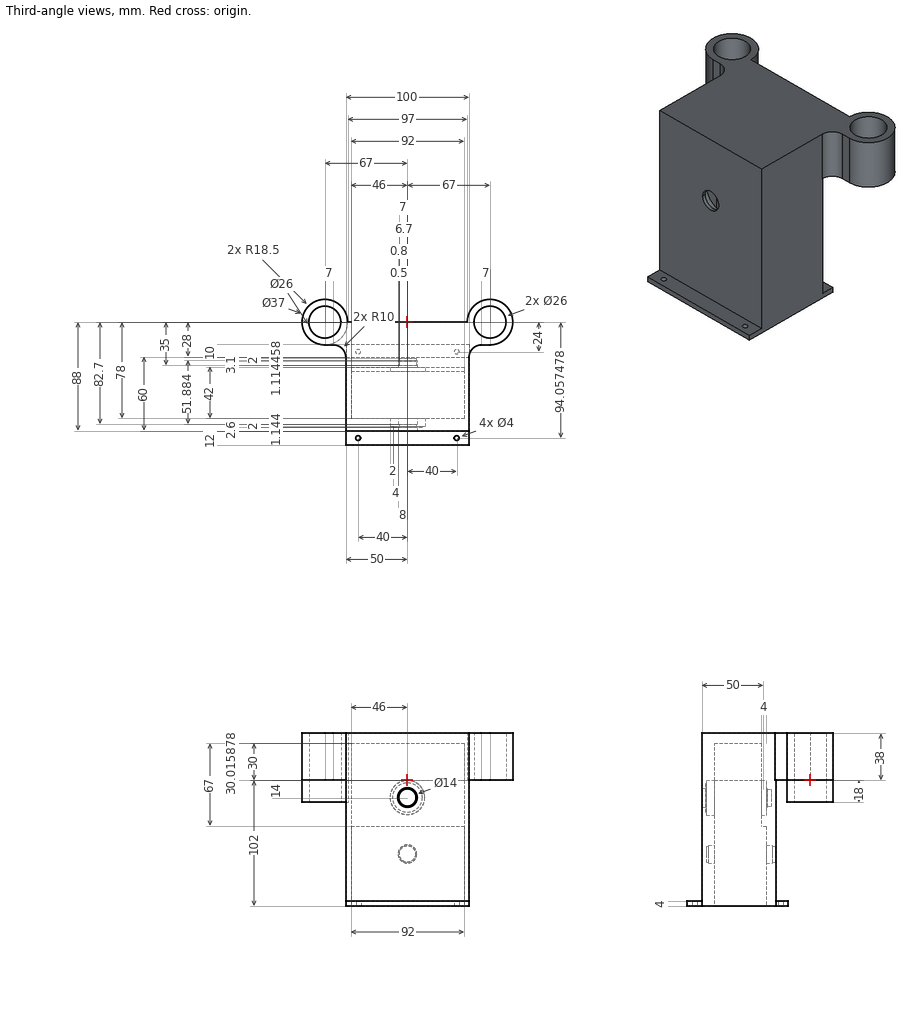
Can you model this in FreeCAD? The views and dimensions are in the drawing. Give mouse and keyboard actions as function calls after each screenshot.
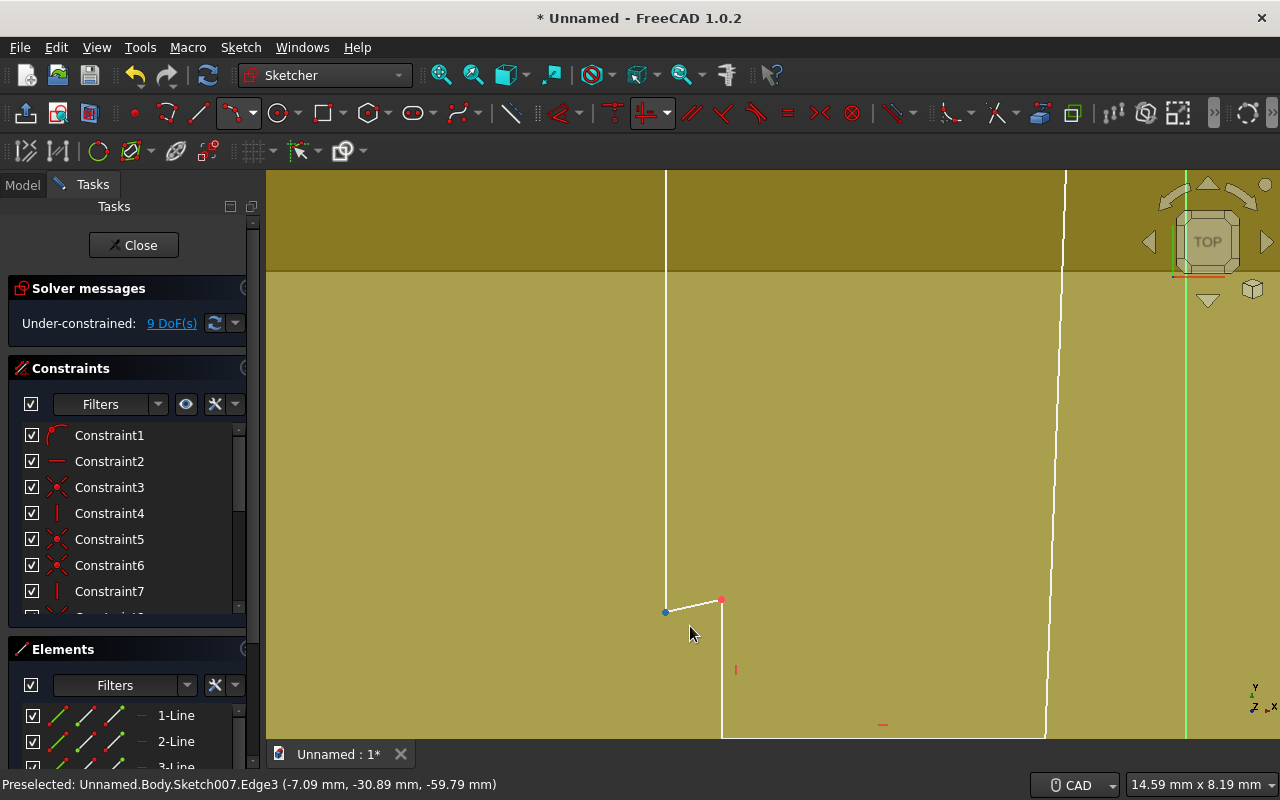
click(683, 608)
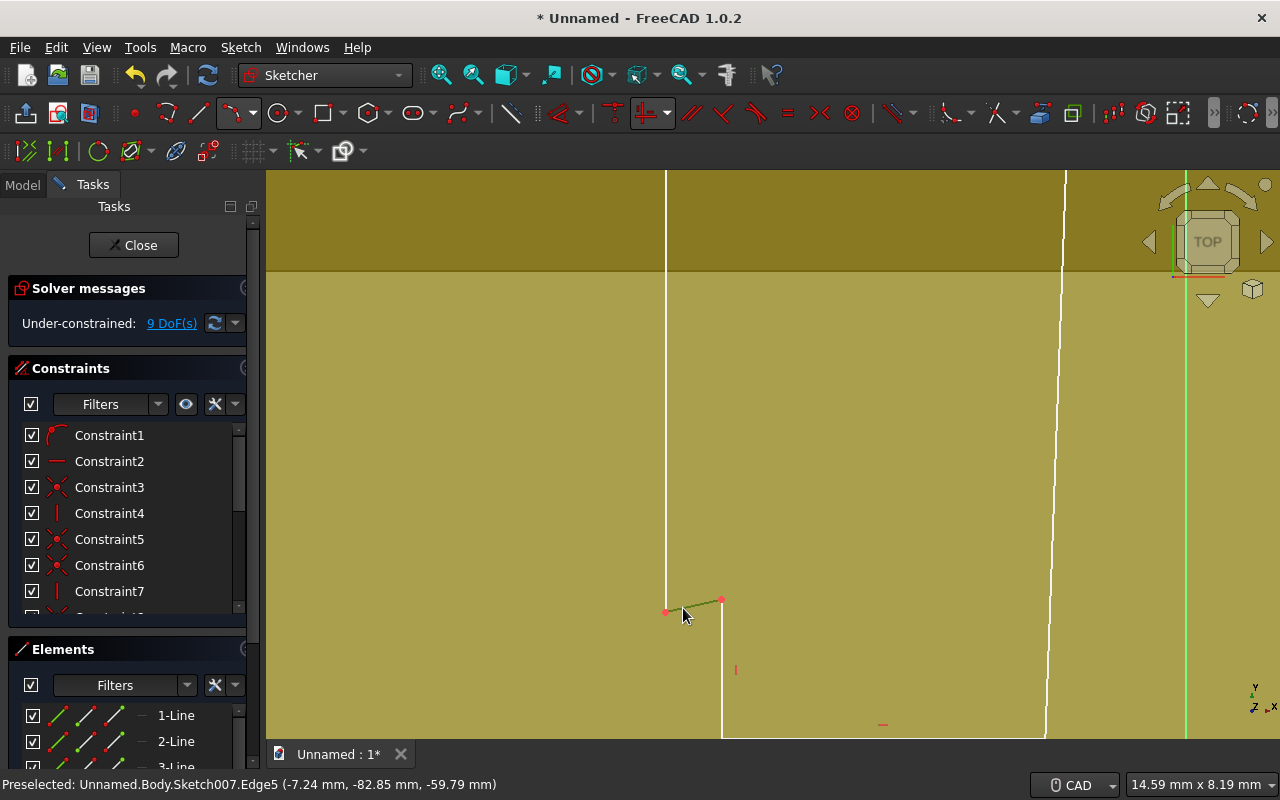
key(h)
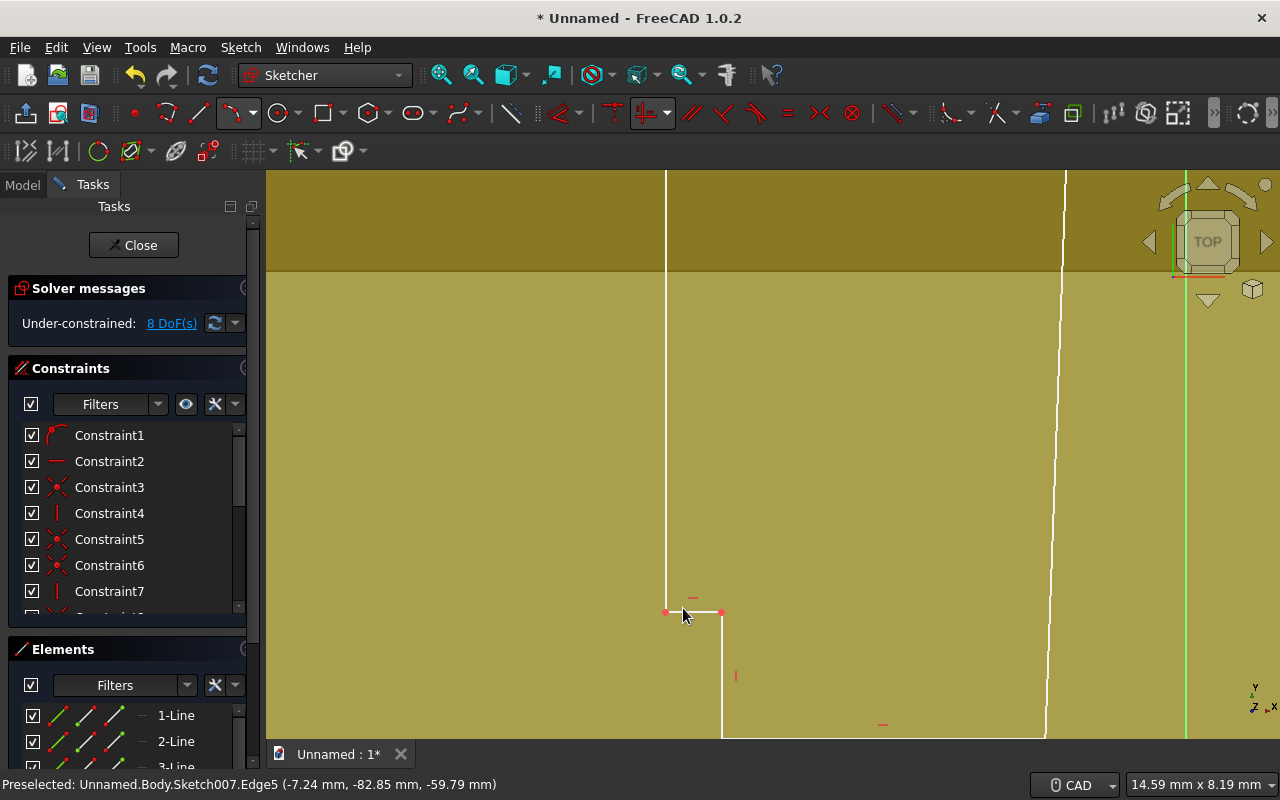
scroll(690, 627, down, 14)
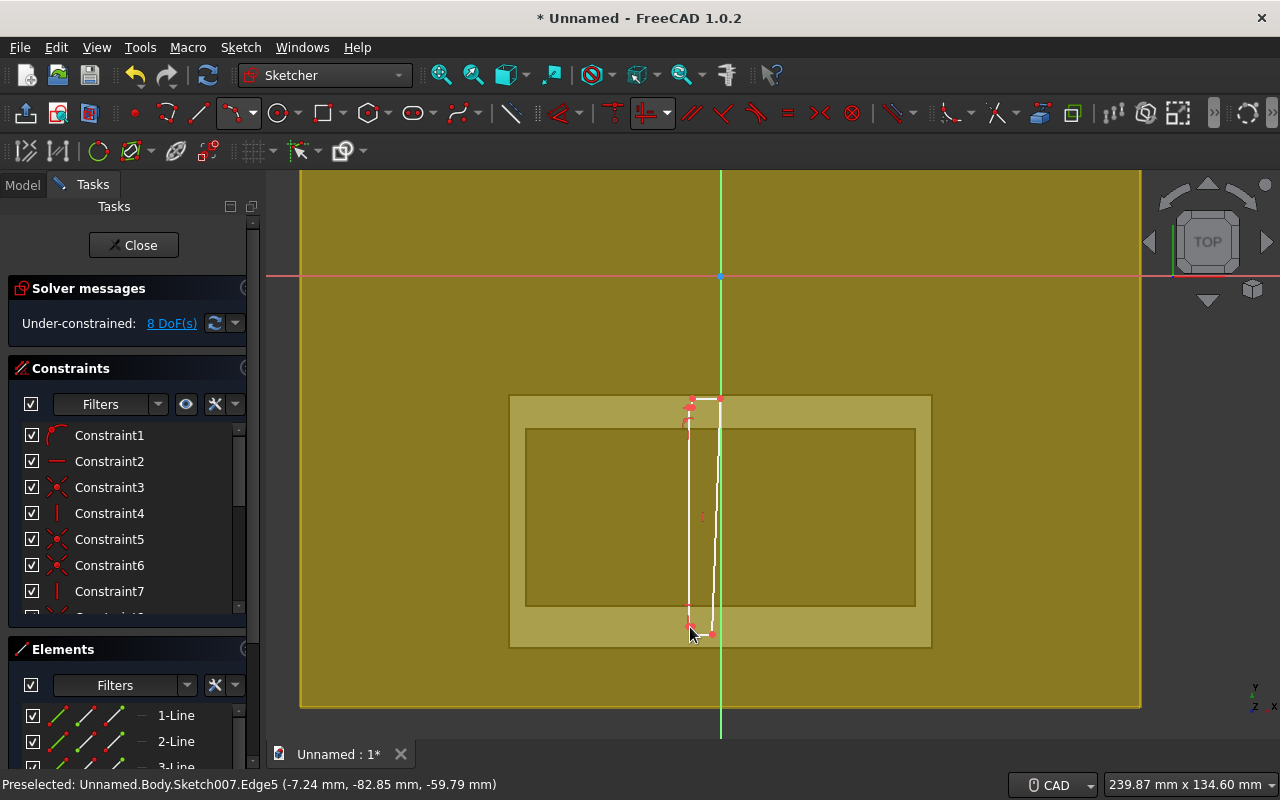
scroll(715, 564, up, 5)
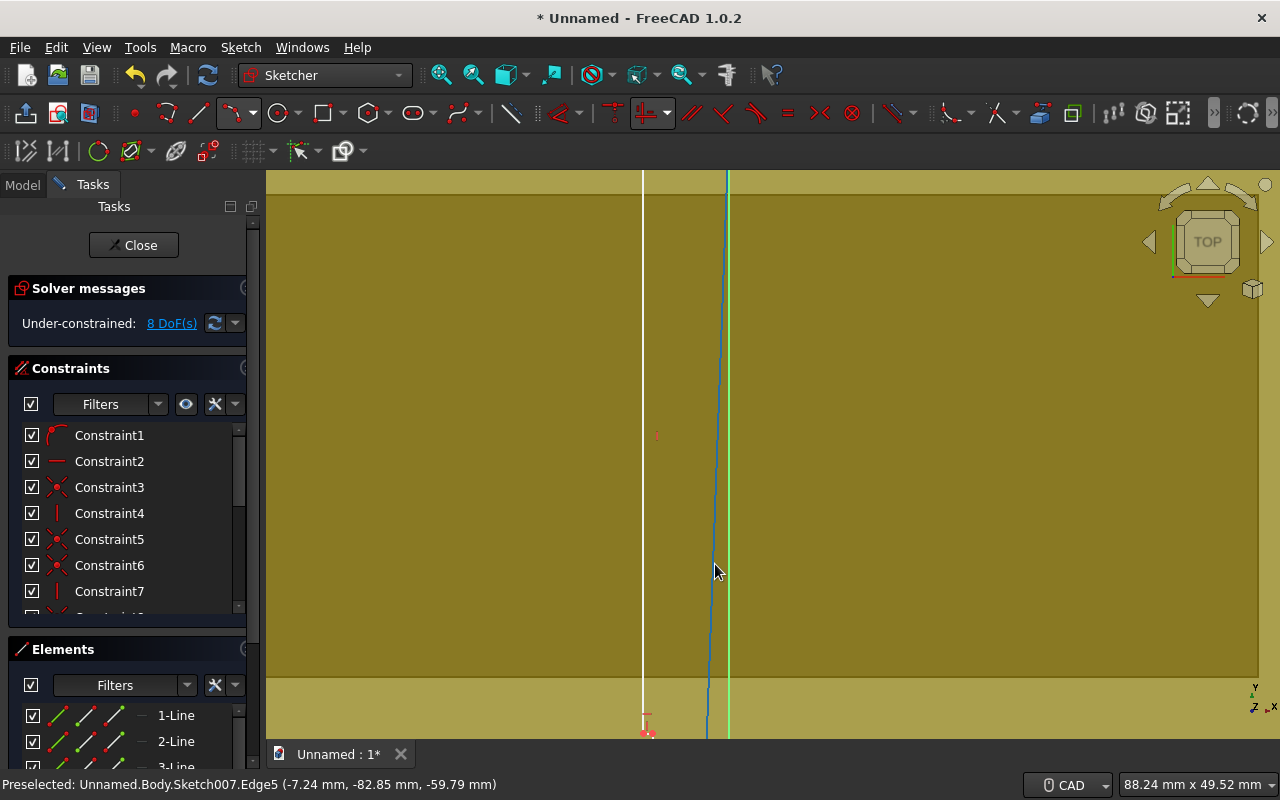
click(713, 562)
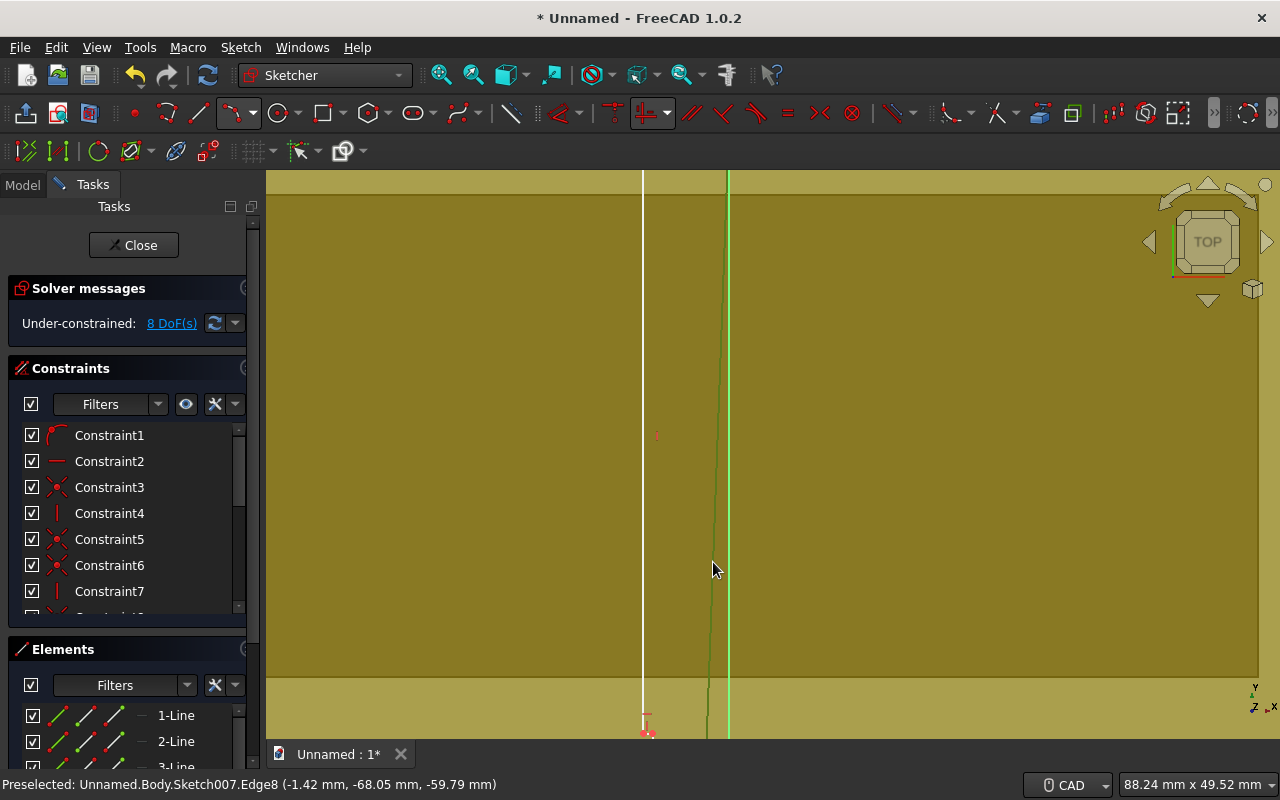
click(670, 114)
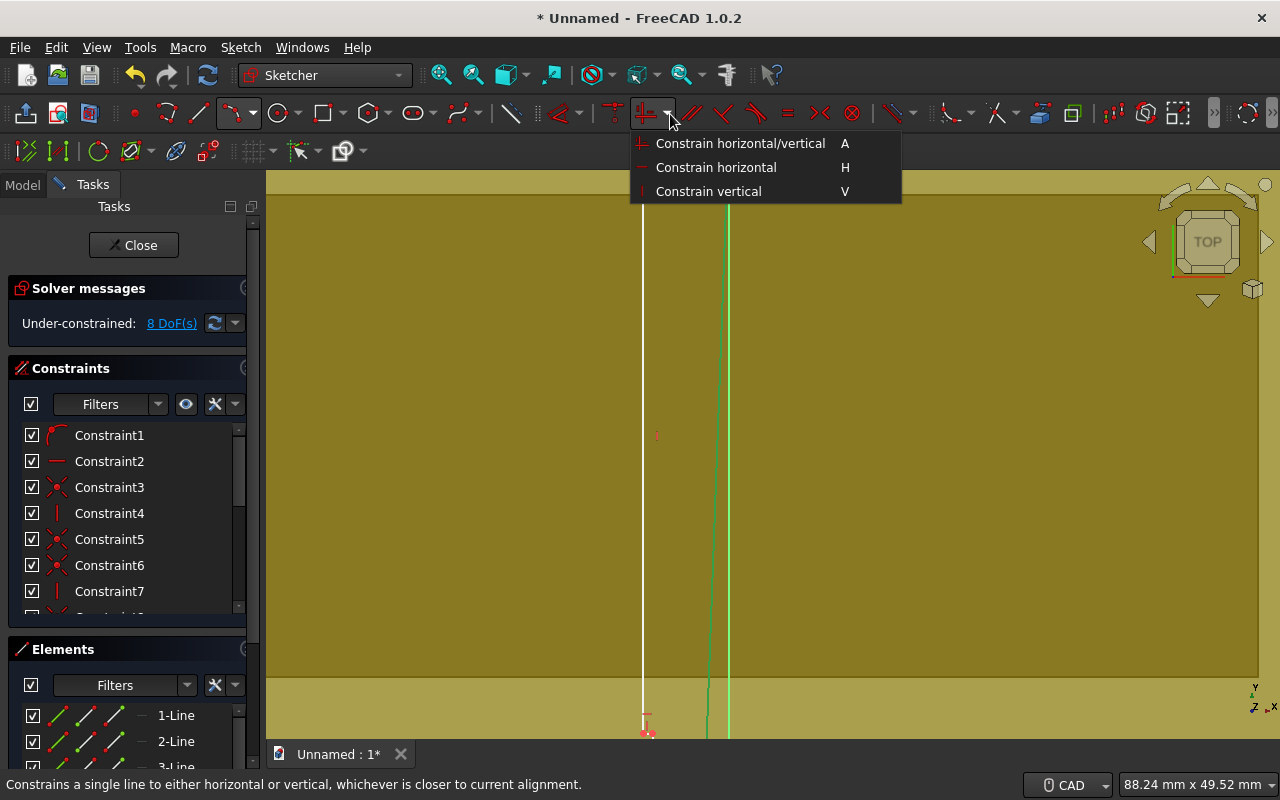
click(766, 191)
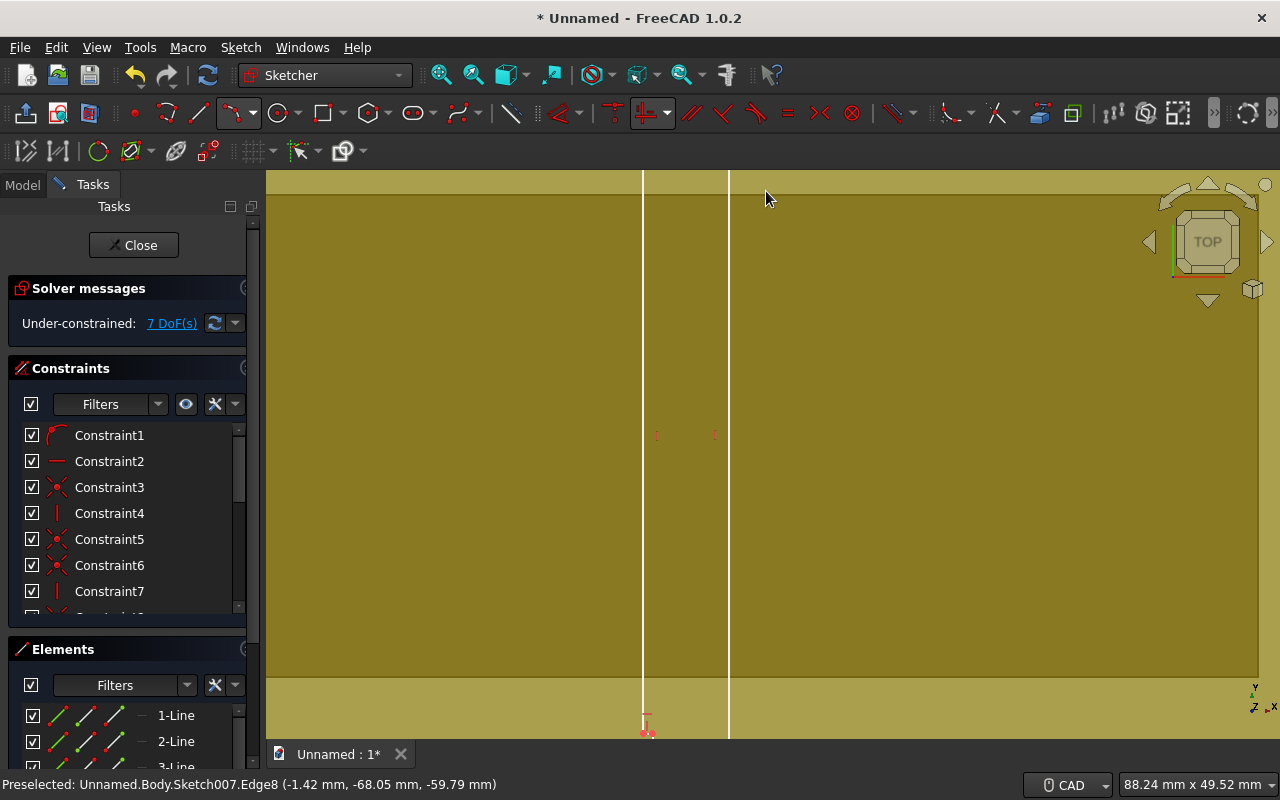
key(d)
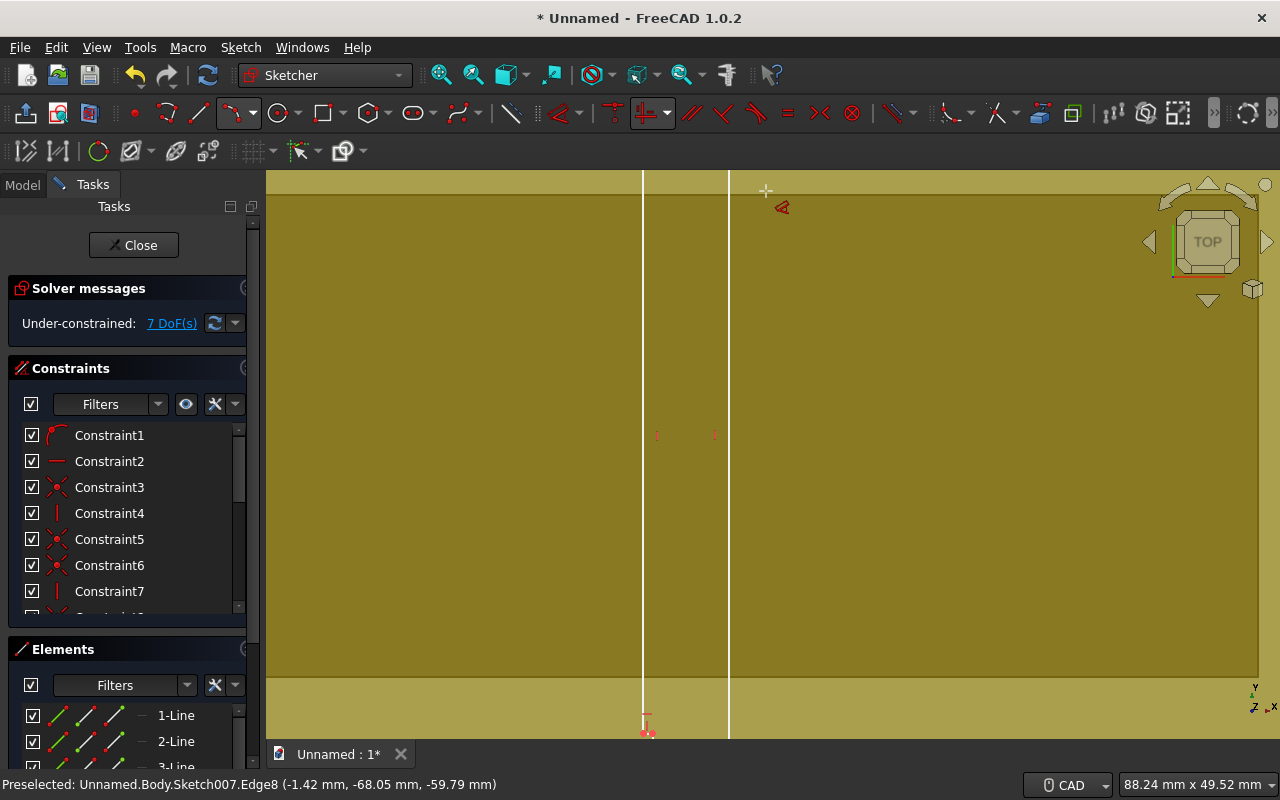
scroll(715, 563, down, 5)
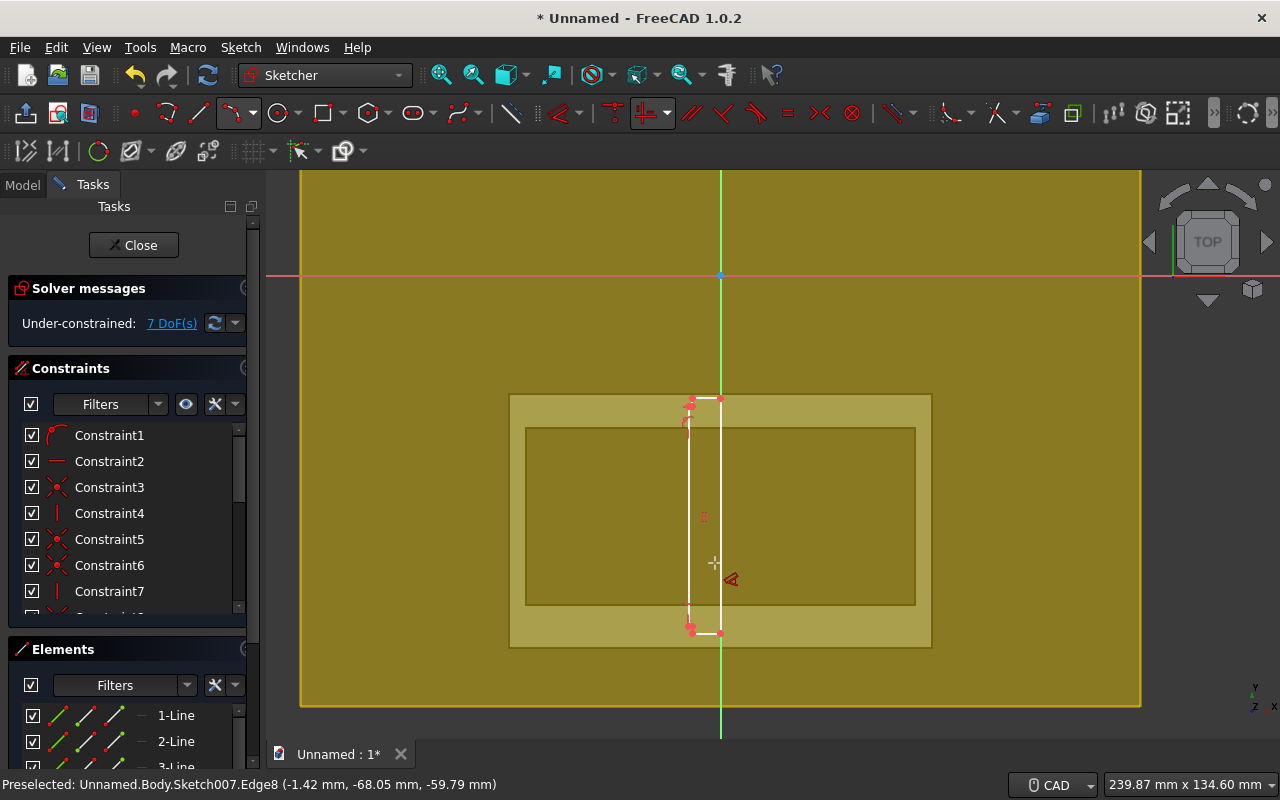
scroll(692, 402, up, 8)